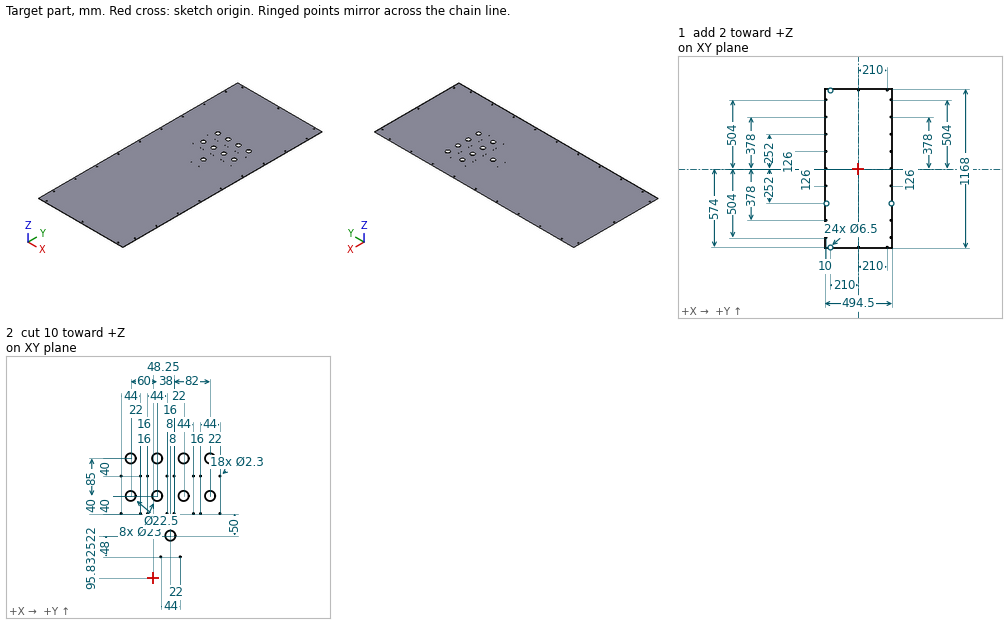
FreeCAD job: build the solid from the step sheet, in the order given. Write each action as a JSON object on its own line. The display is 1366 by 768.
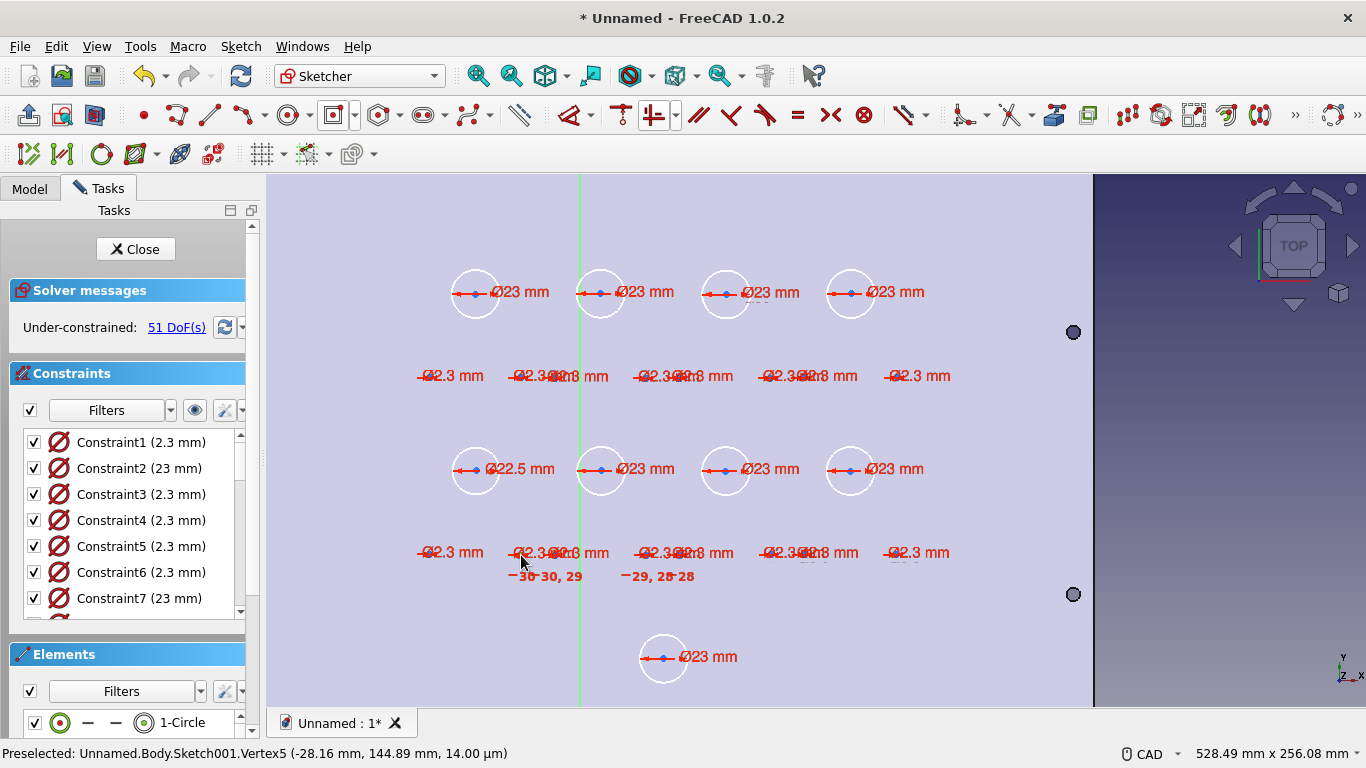
{"action": "left_click", "coordinate": [430, 554]}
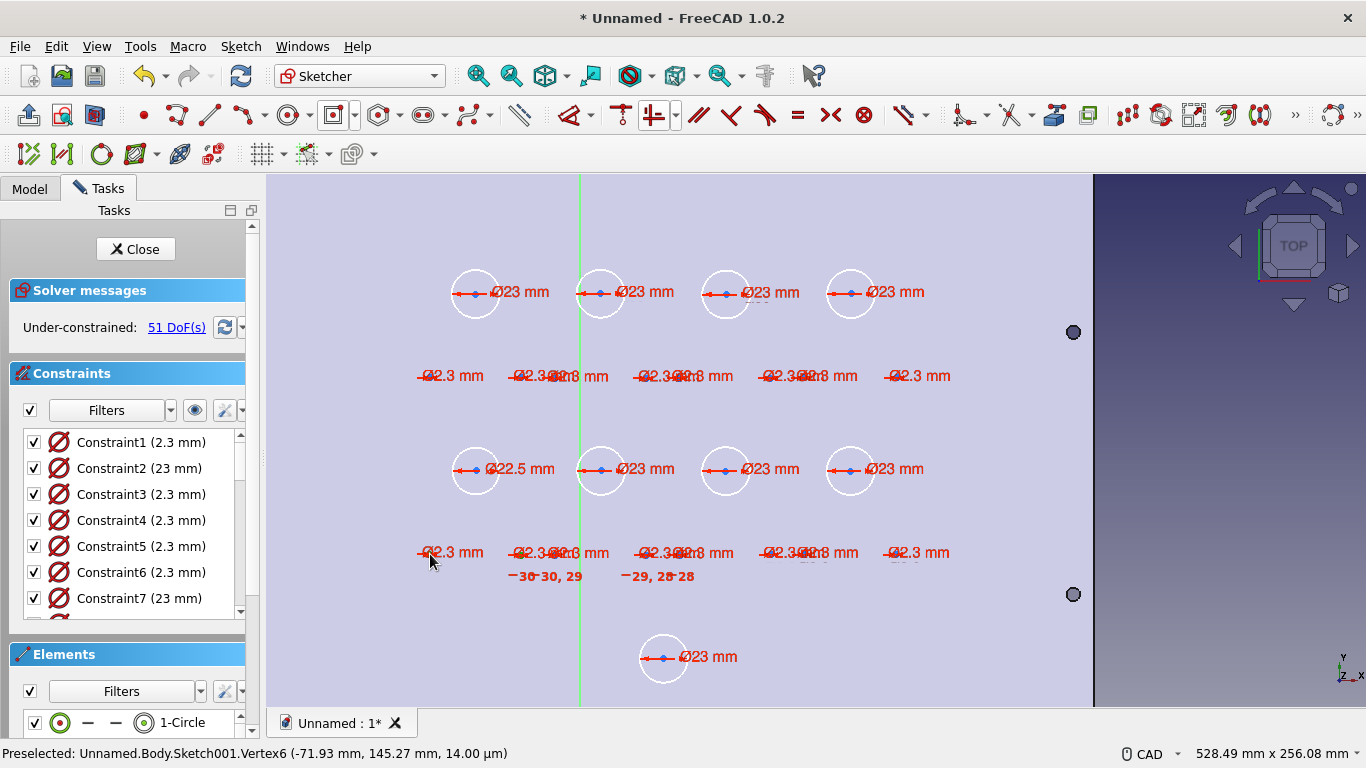
{"action": "key", "text": "h"}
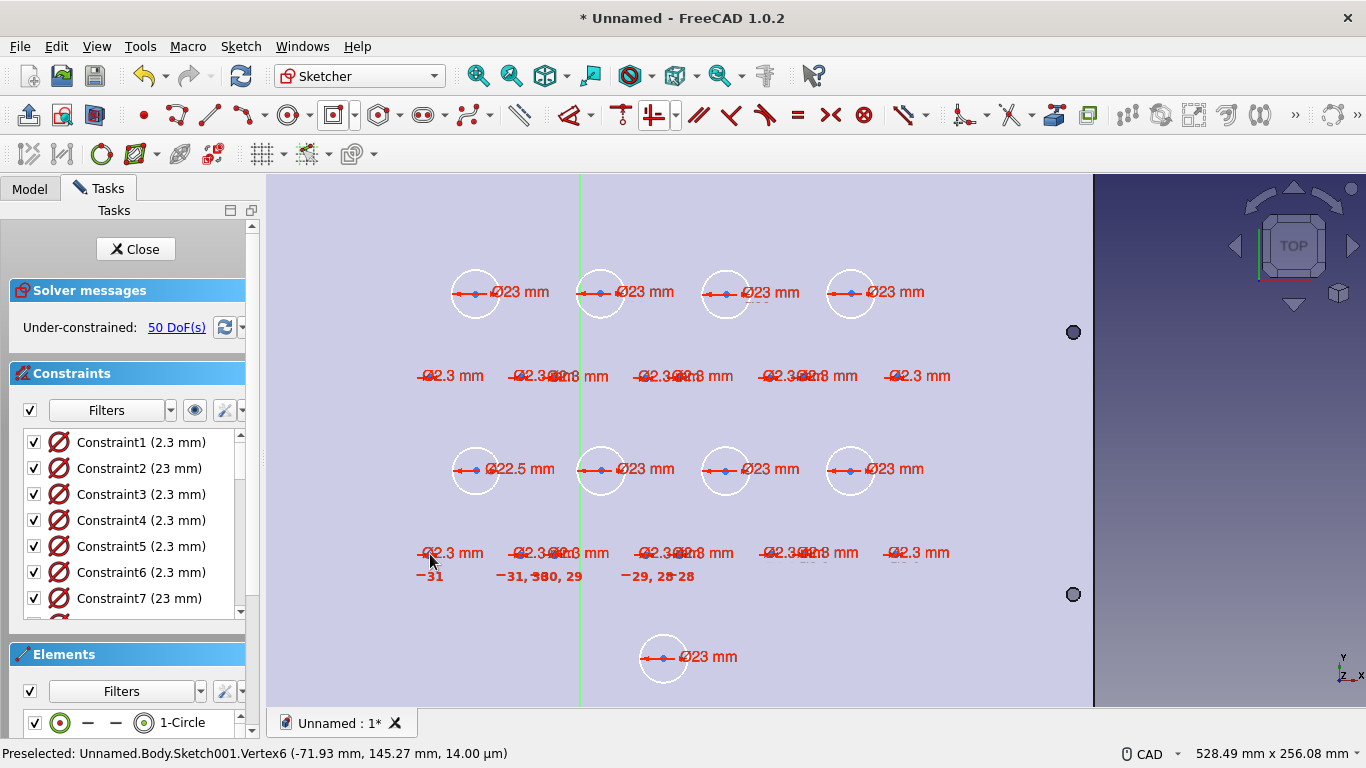
{"action": "left_click", "coordinate": [521, 555]}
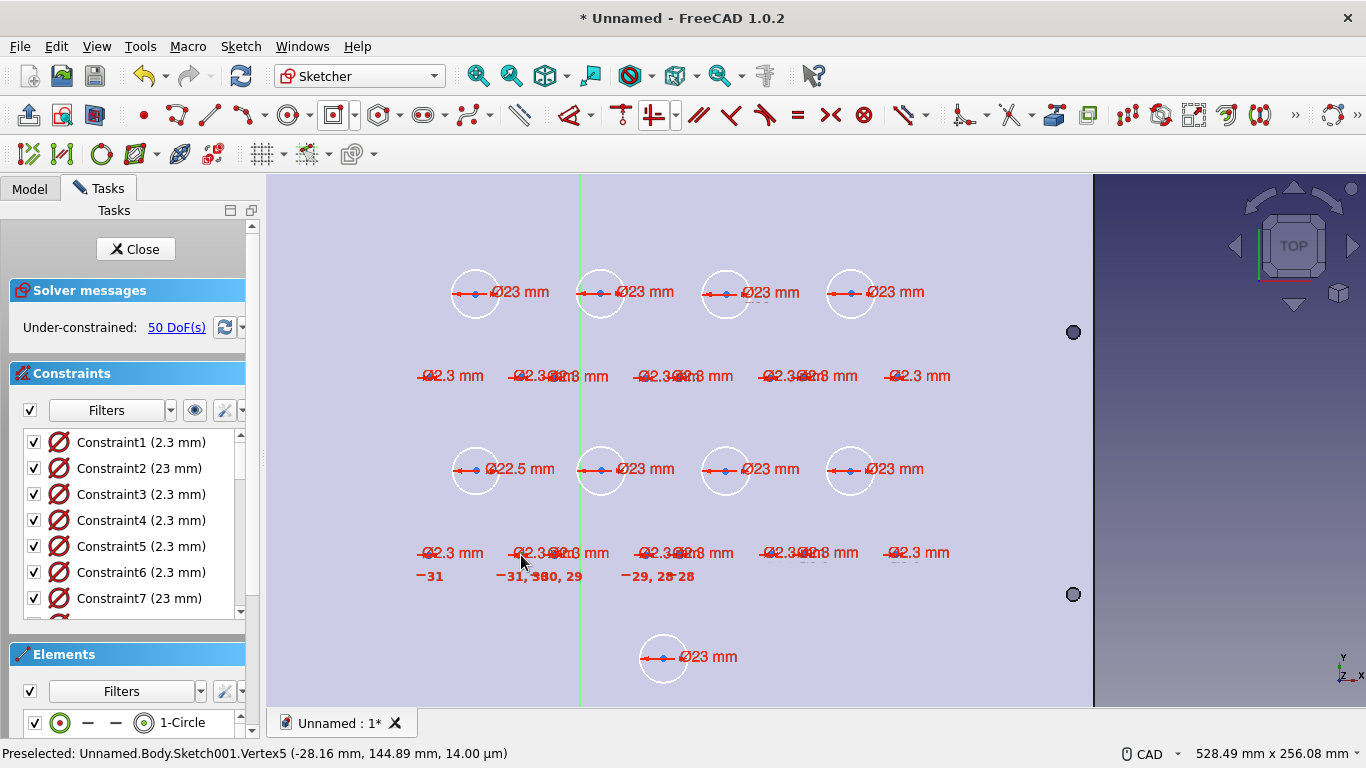
{"action": "left_click", "coordinate": [521, 378]}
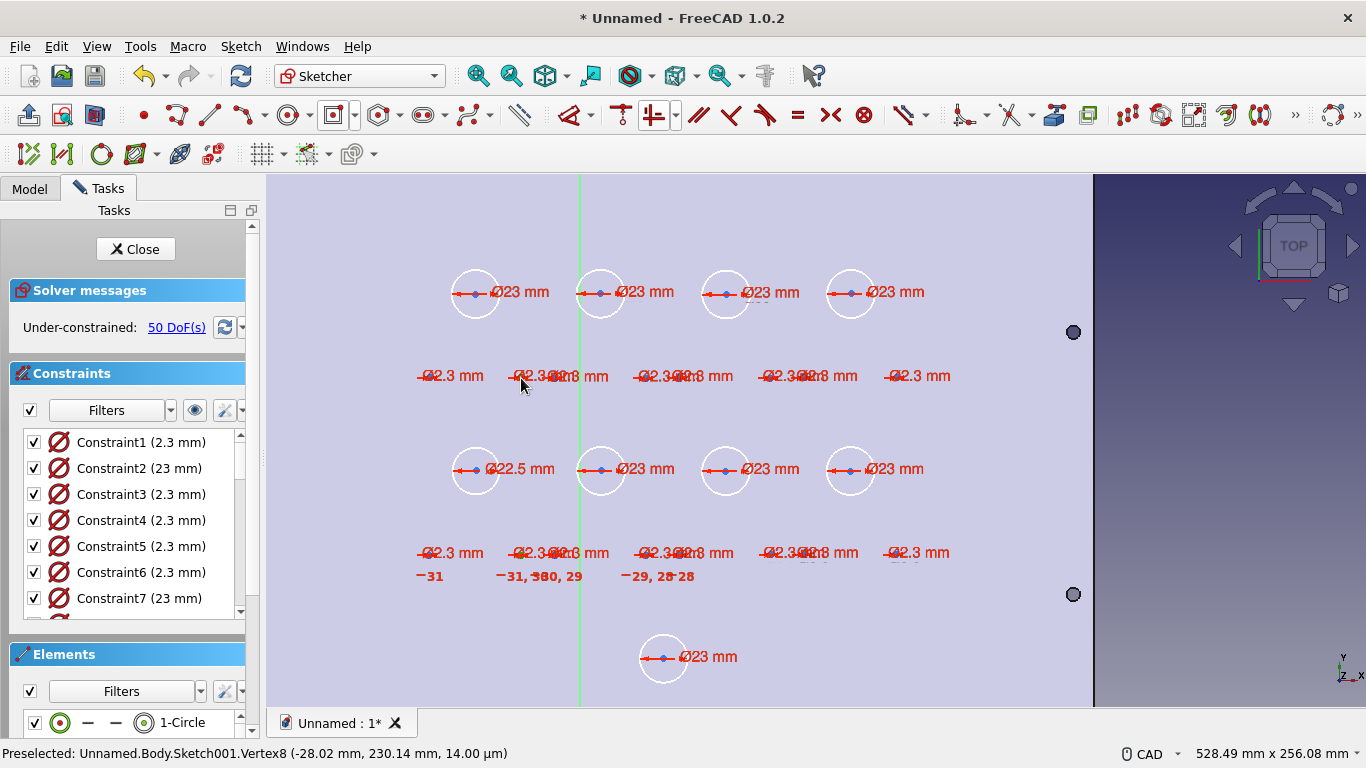
{"action": "left_click", "coordinate": [676, 116]}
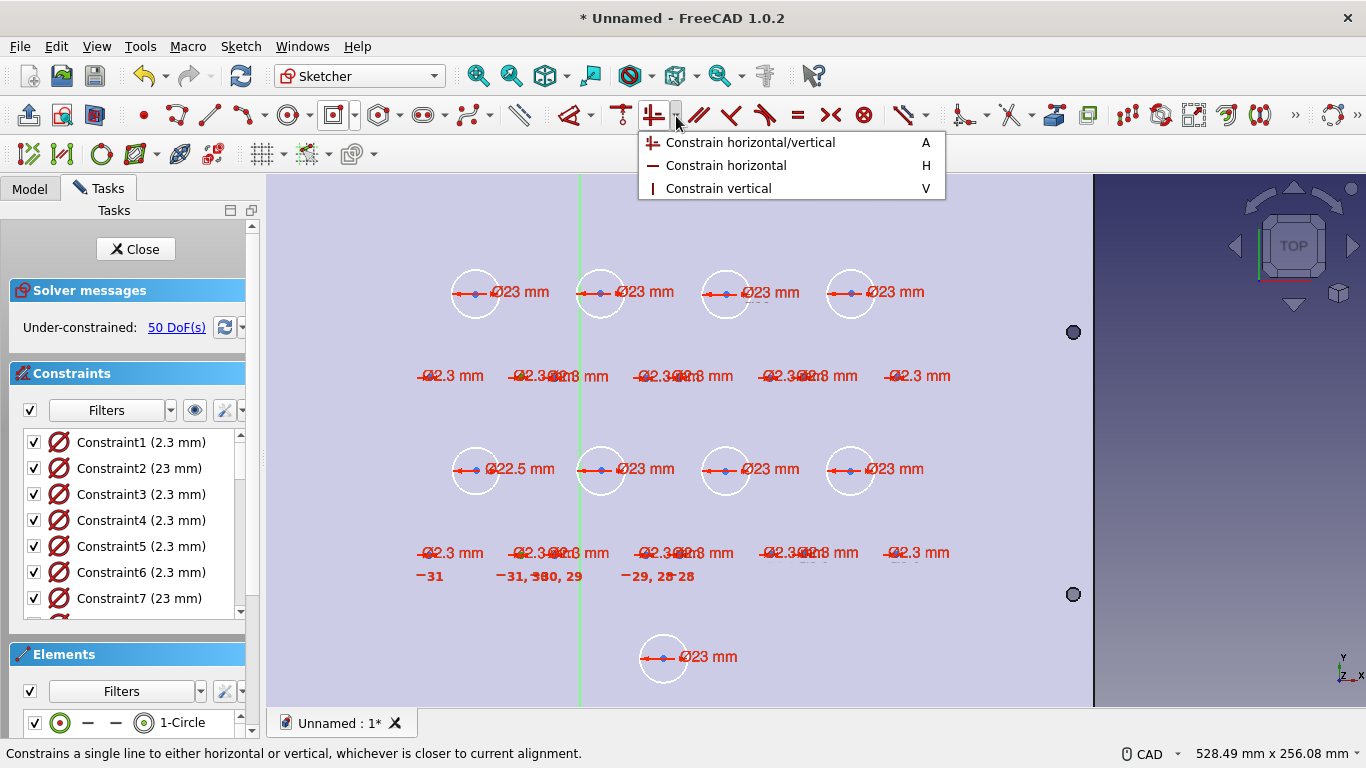
{"action": "left_click", "coordinate": [792, 188]}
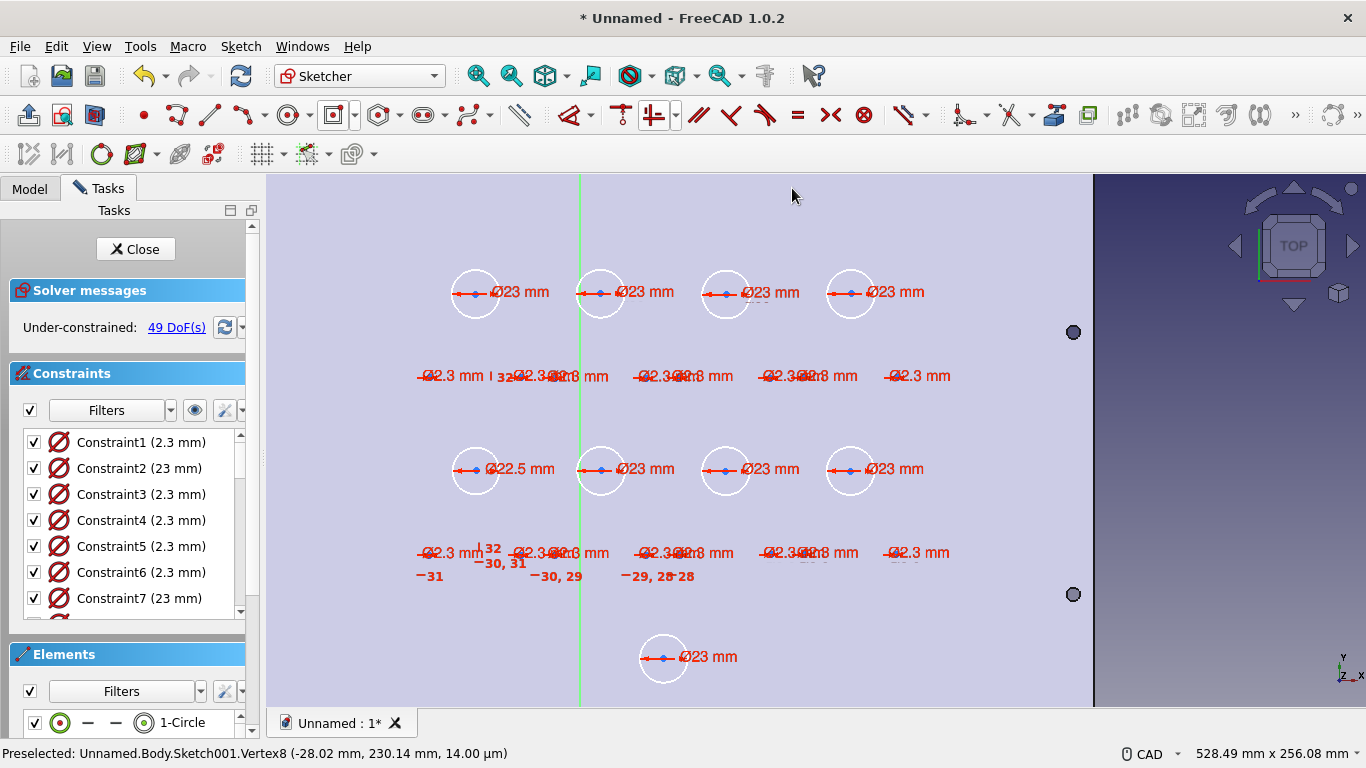
{"action": "left_click", "coordinate": [430, 555]}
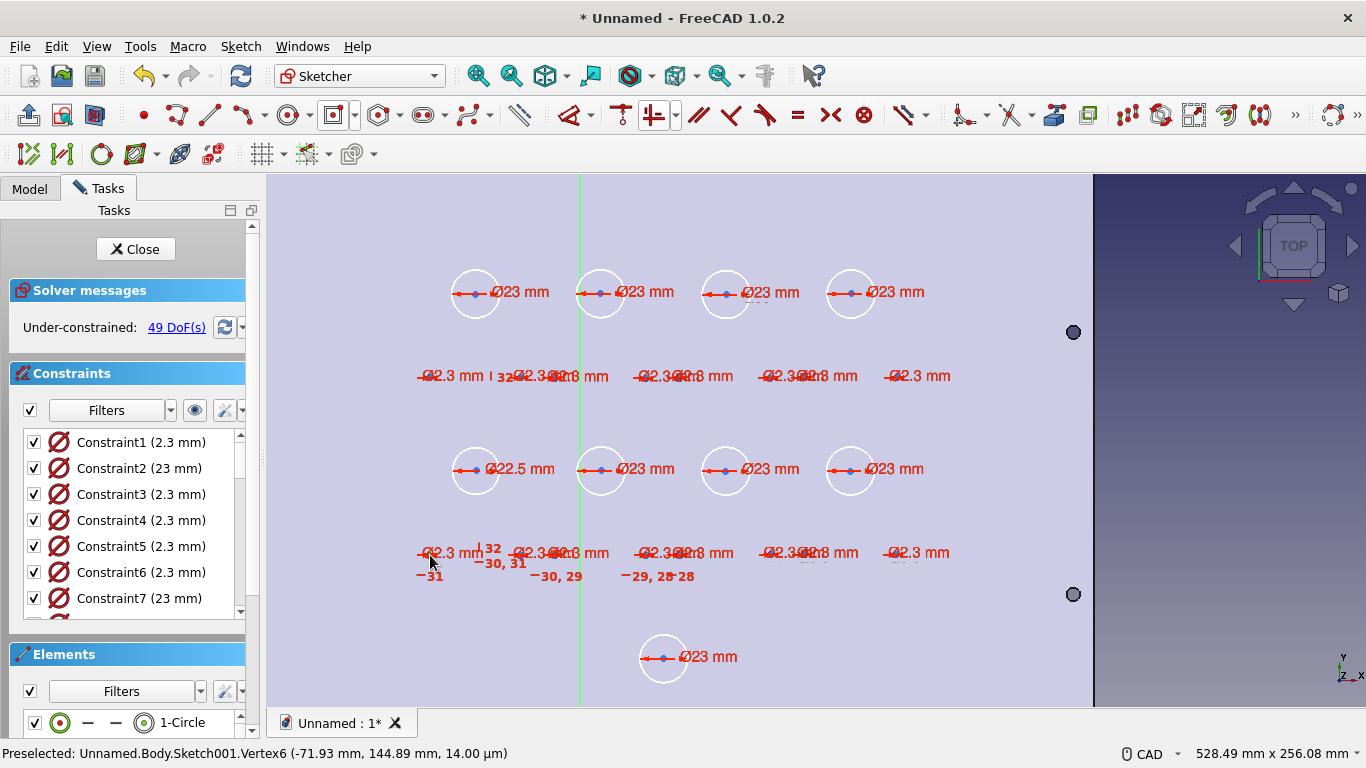
{"action": "left_click", "coordinate": [430, 378]}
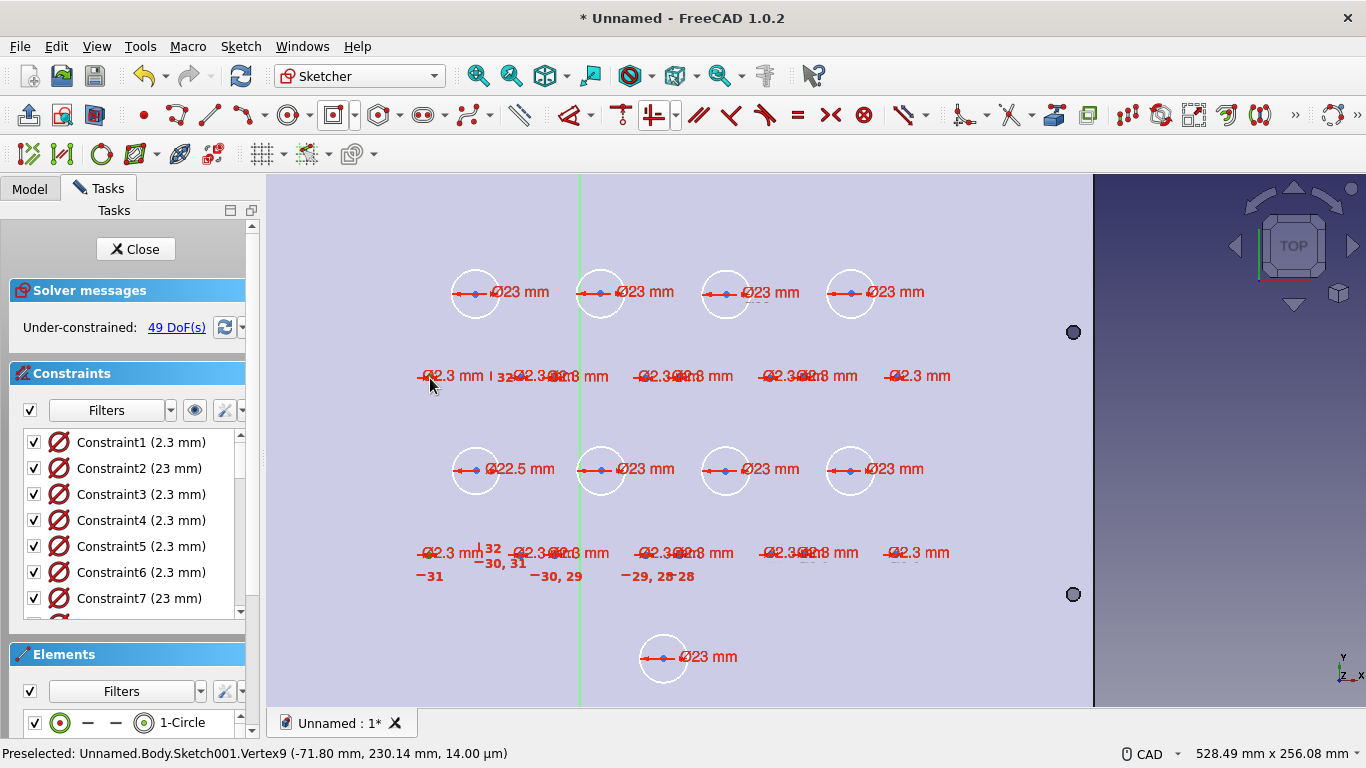
{"action": "left_click", "coordinate": [676, 116]}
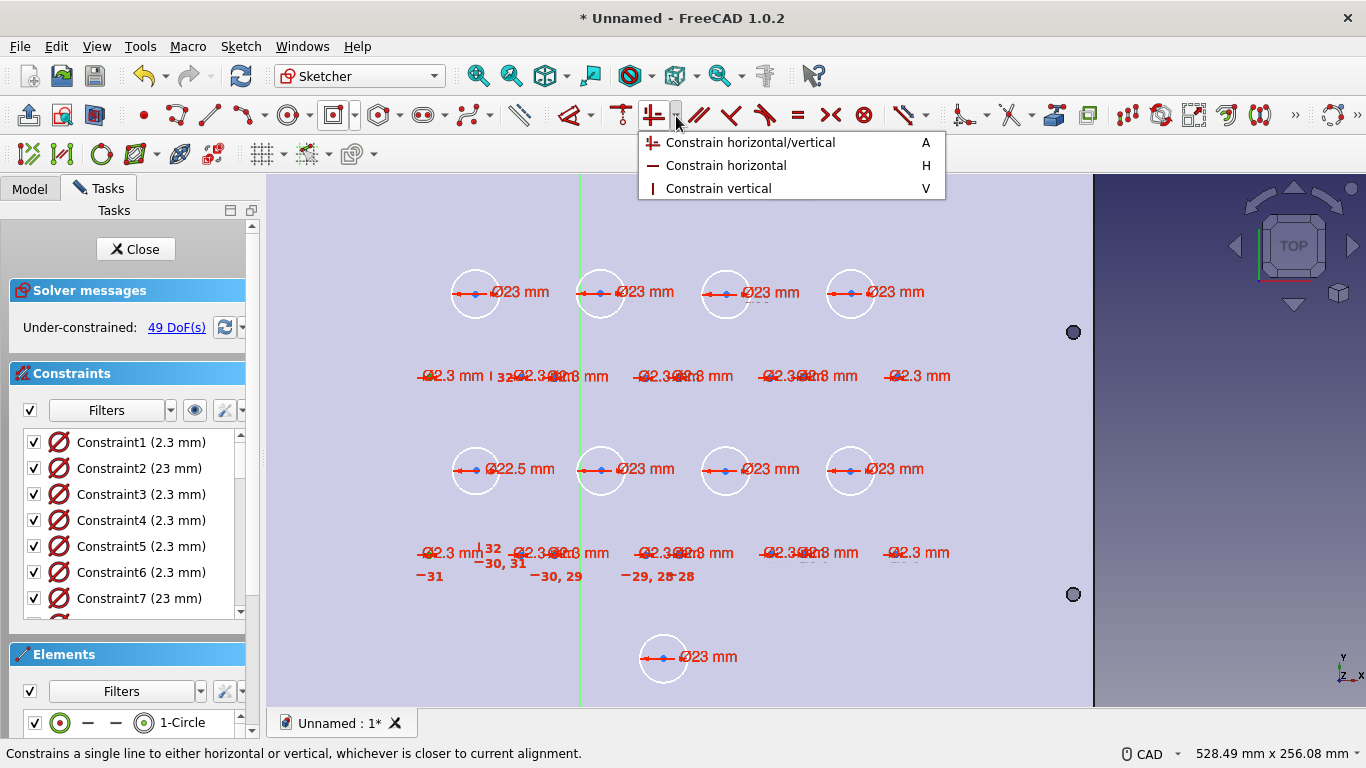
{"action": "left_click", "coordinate": [792, 188]}